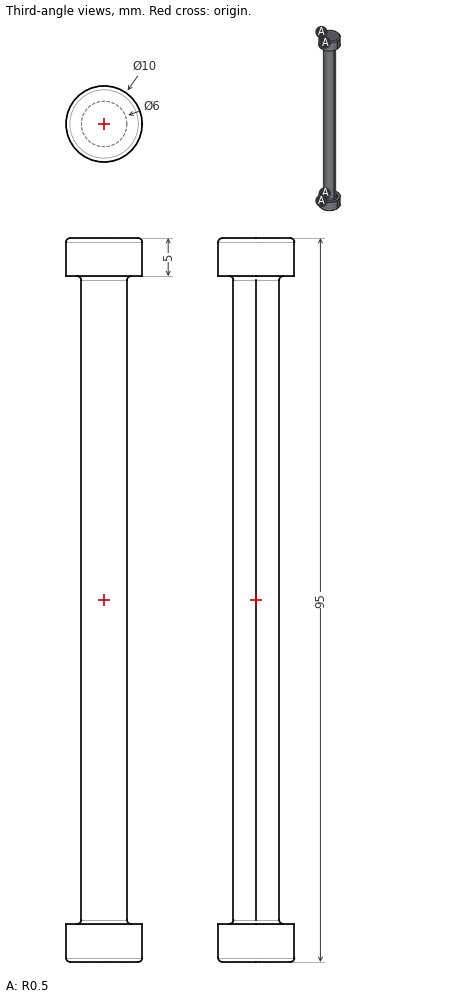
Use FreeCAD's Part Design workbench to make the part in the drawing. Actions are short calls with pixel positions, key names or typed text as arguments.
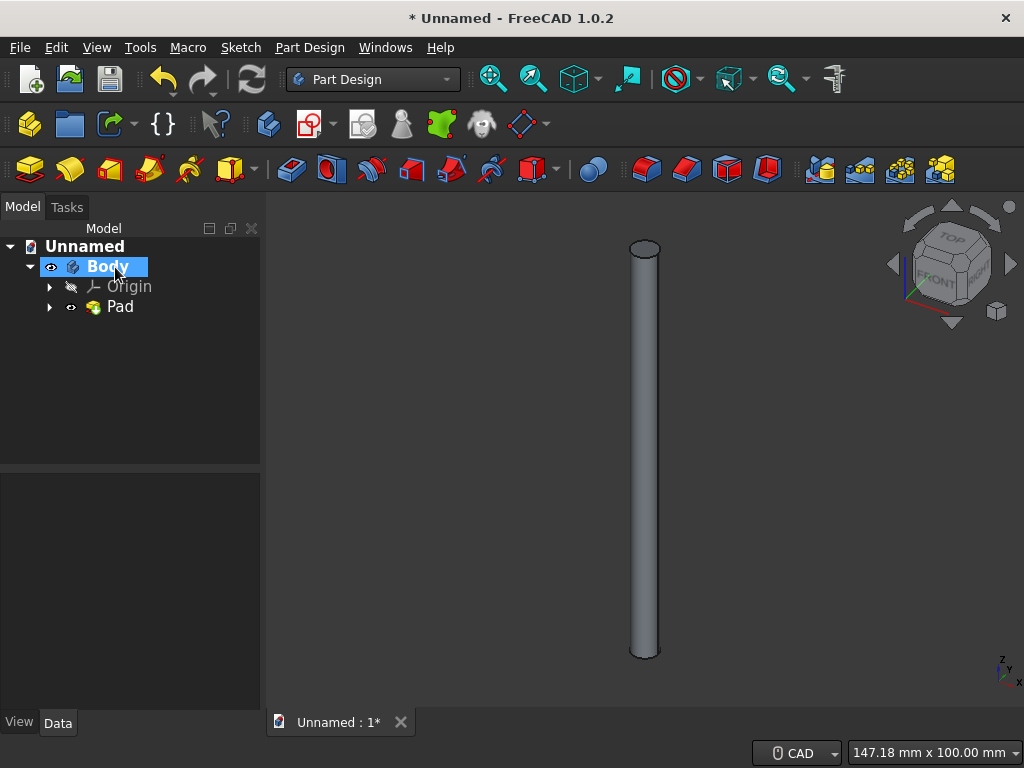
click(645, 248)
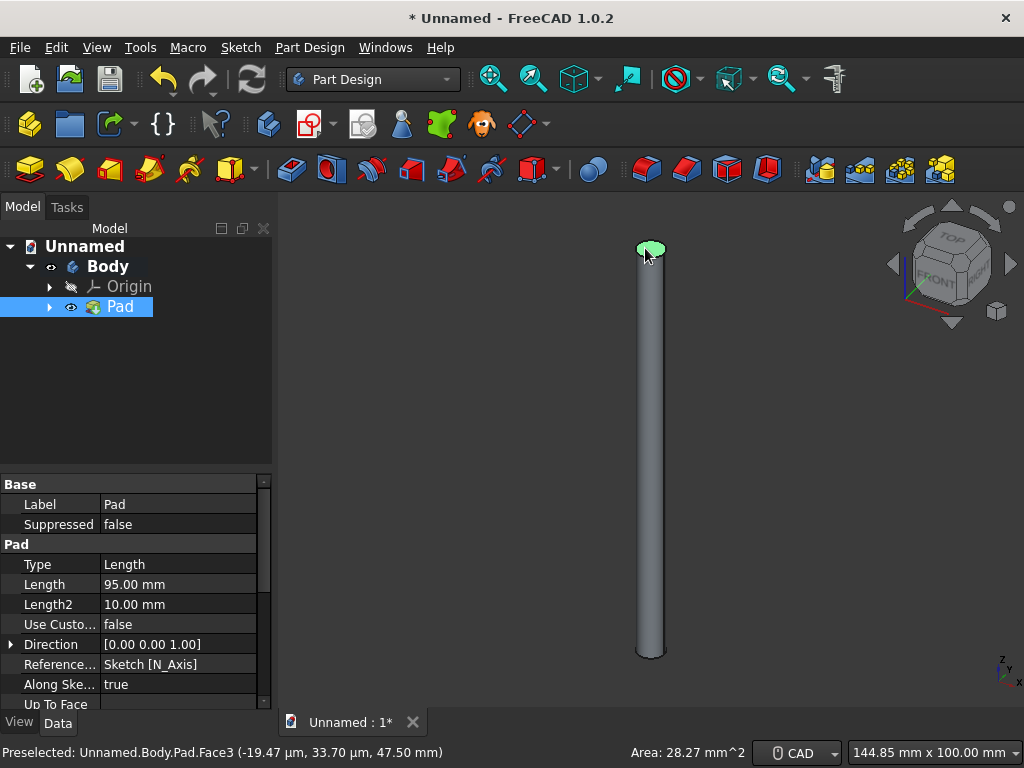
click(310, 124)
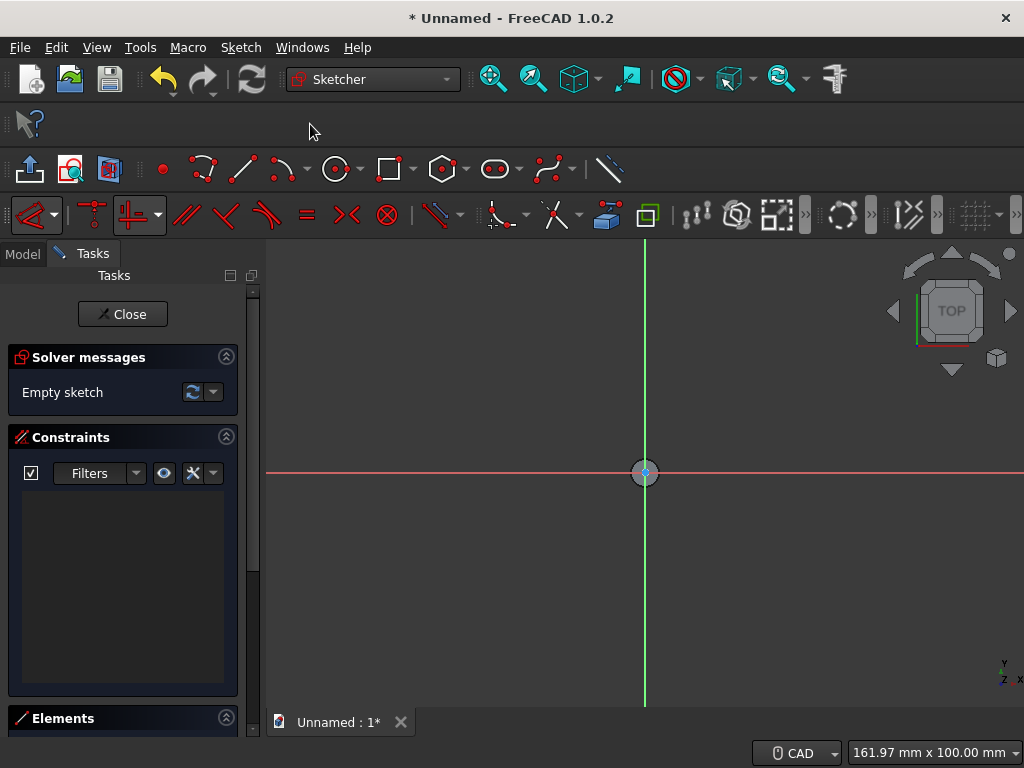
scroll(659, 473, up, 9)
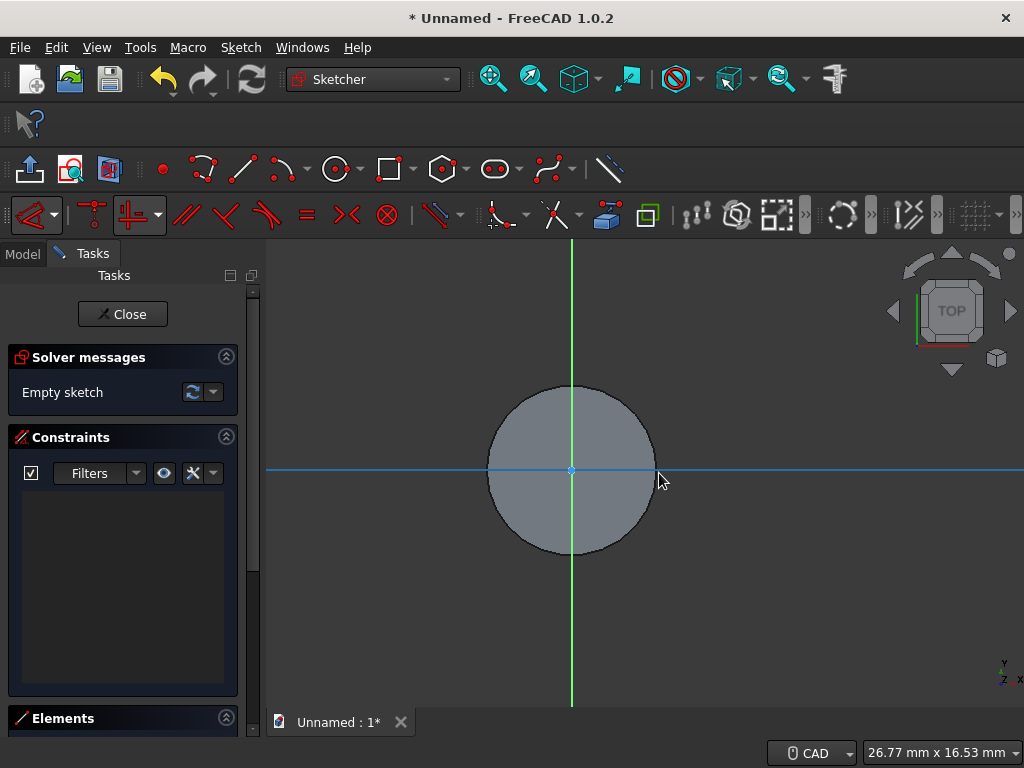
click(336, 170)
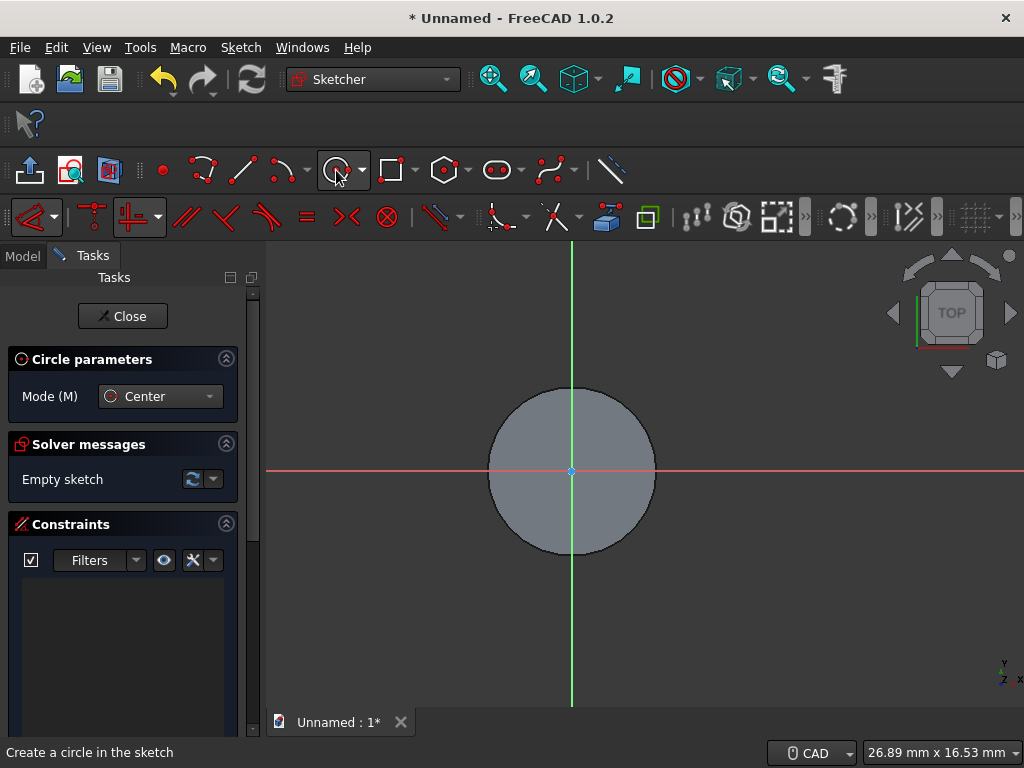
click(572, 471)
move(672, 372)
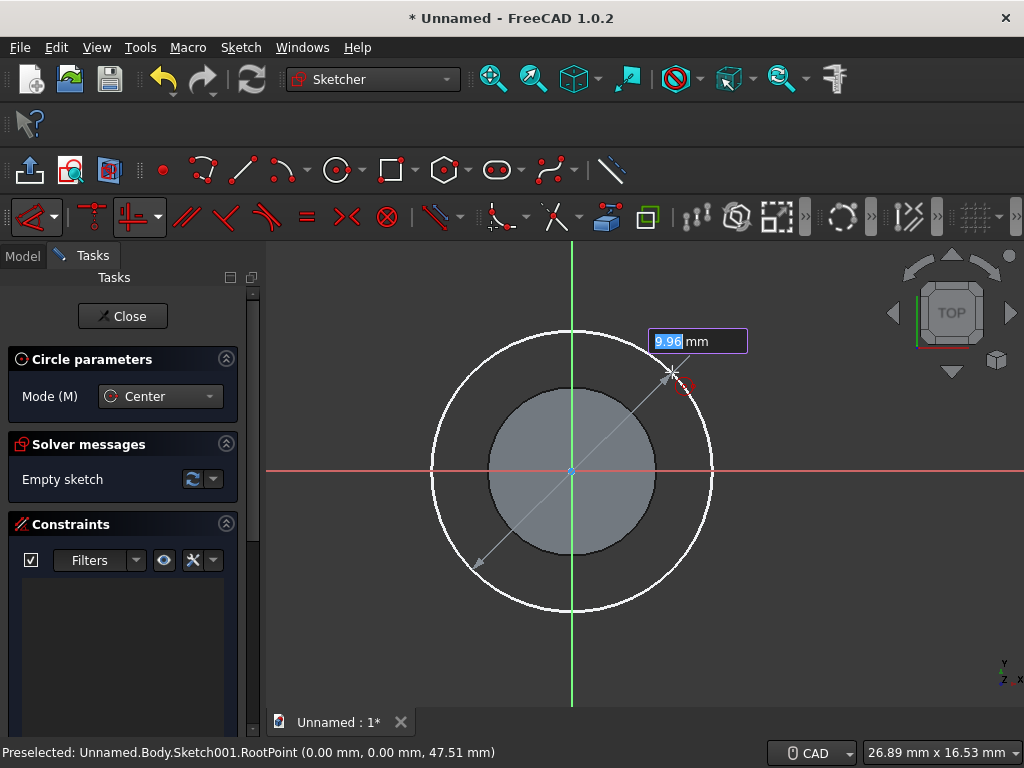
text(10)
key(Return)
key(Escape)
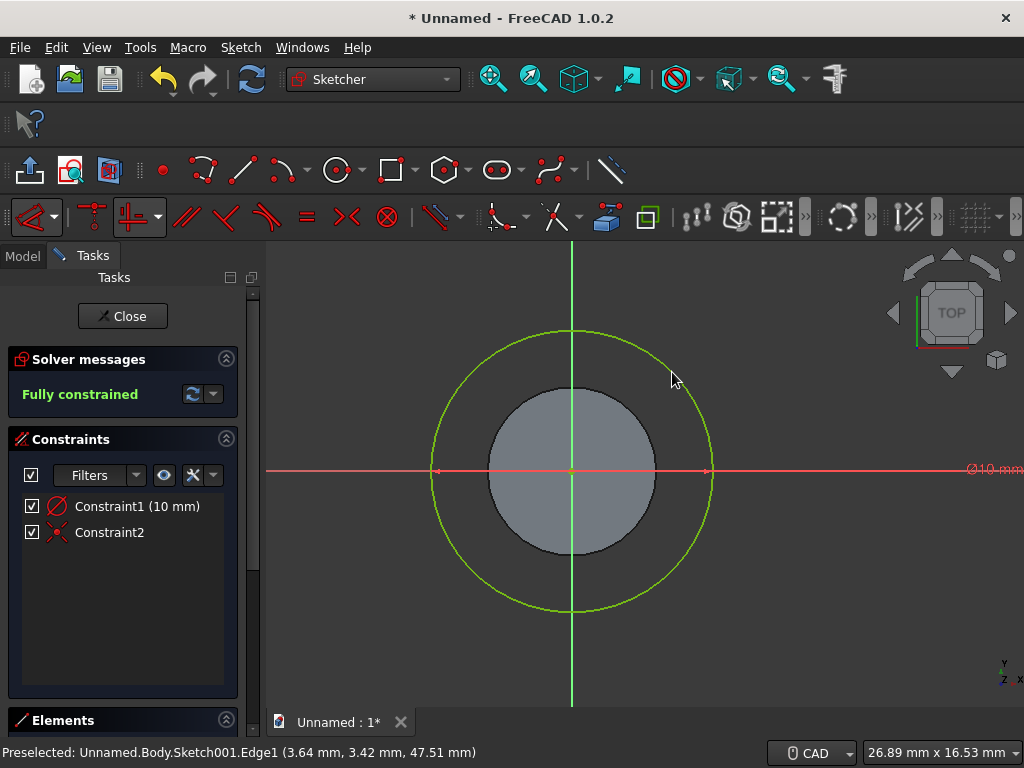
click(123, 316)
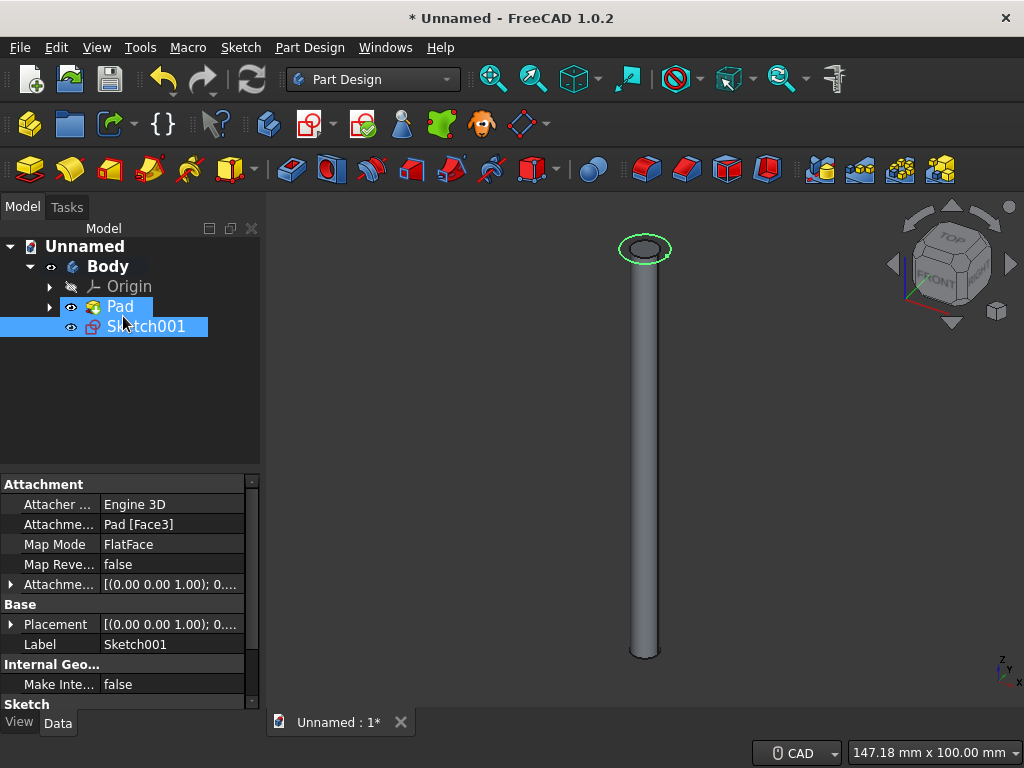
click(30, 170)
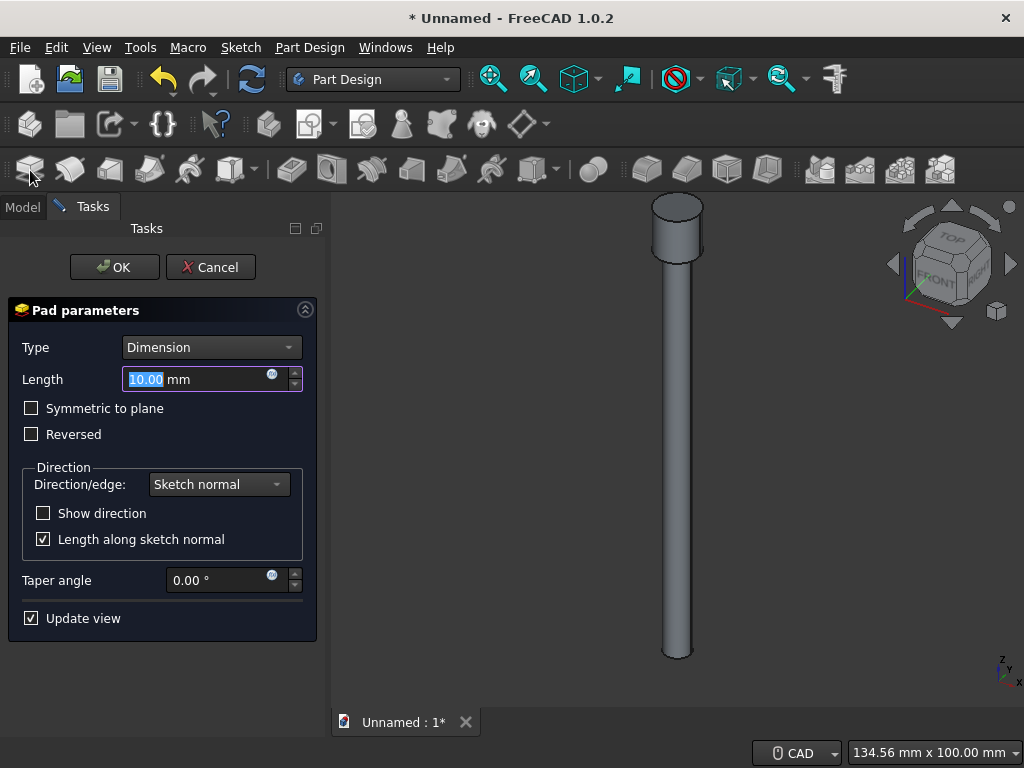
text(5)
key(Tab)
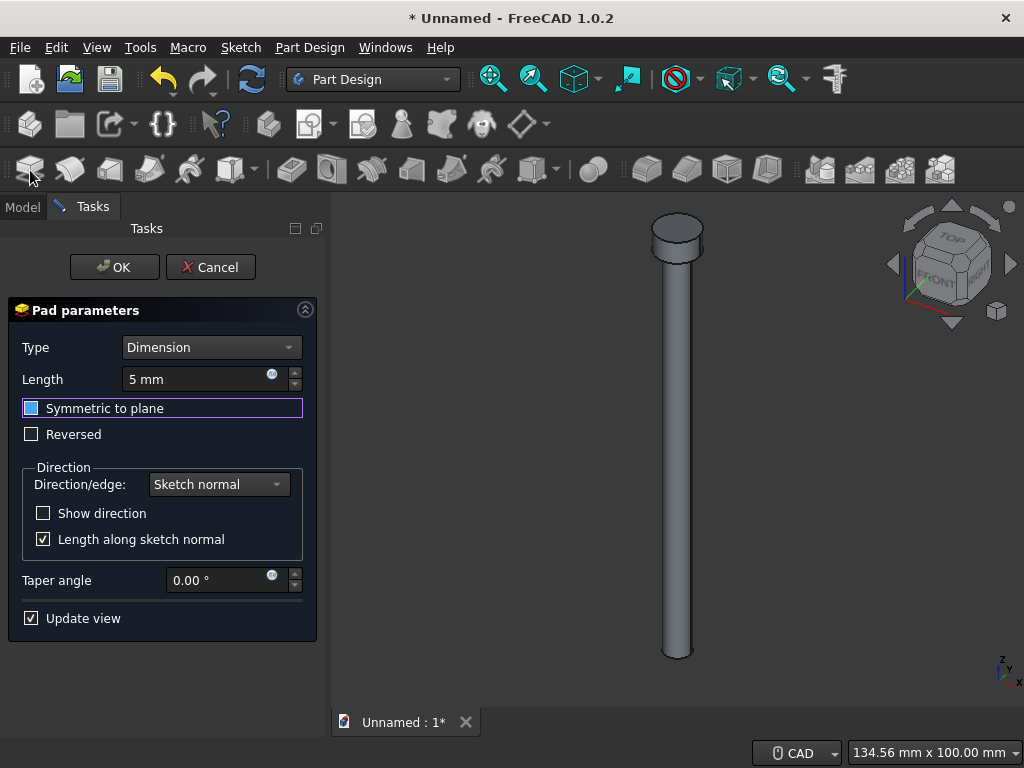
click(30, 434)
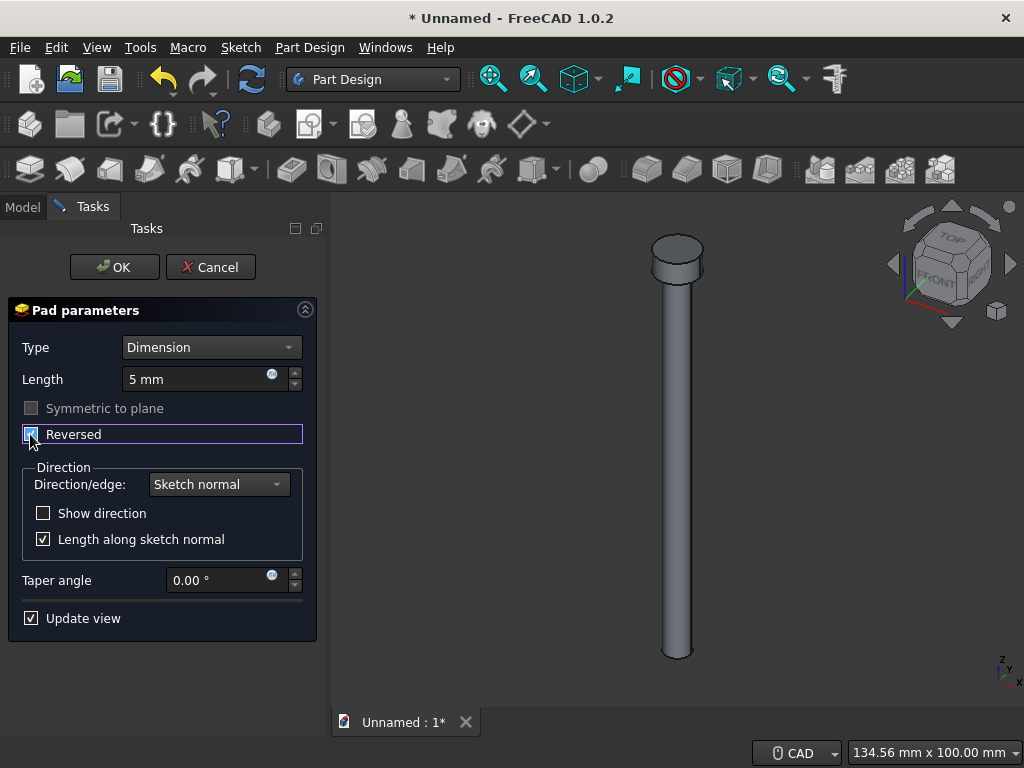
click(115, 267)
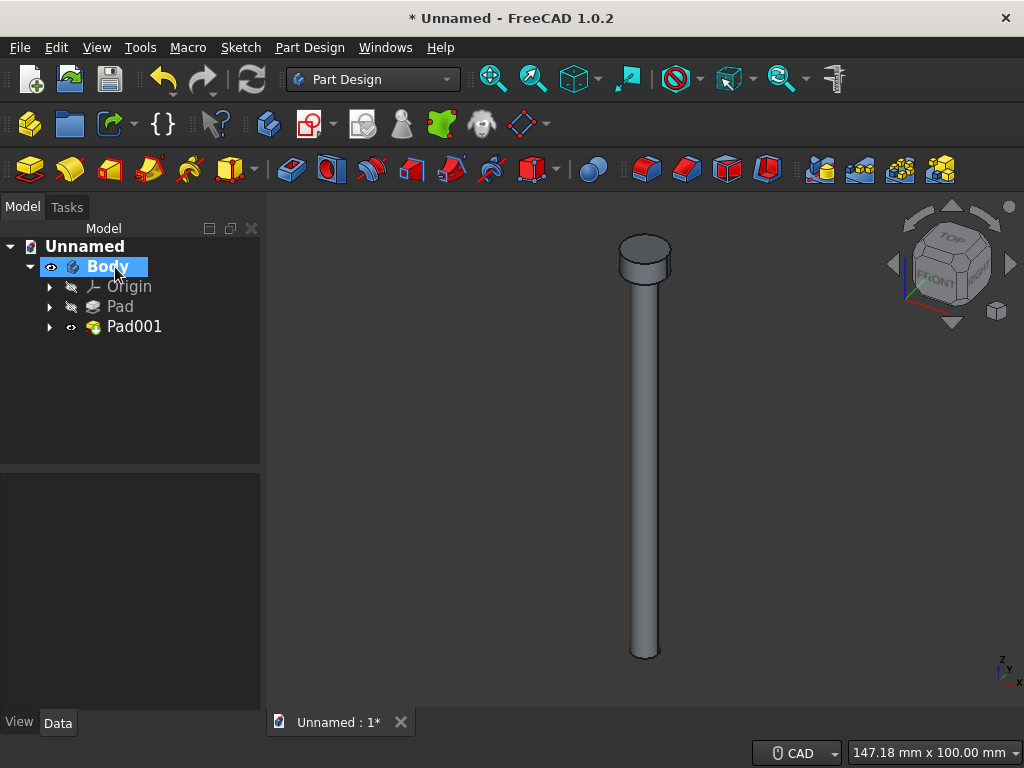
click(116, 327)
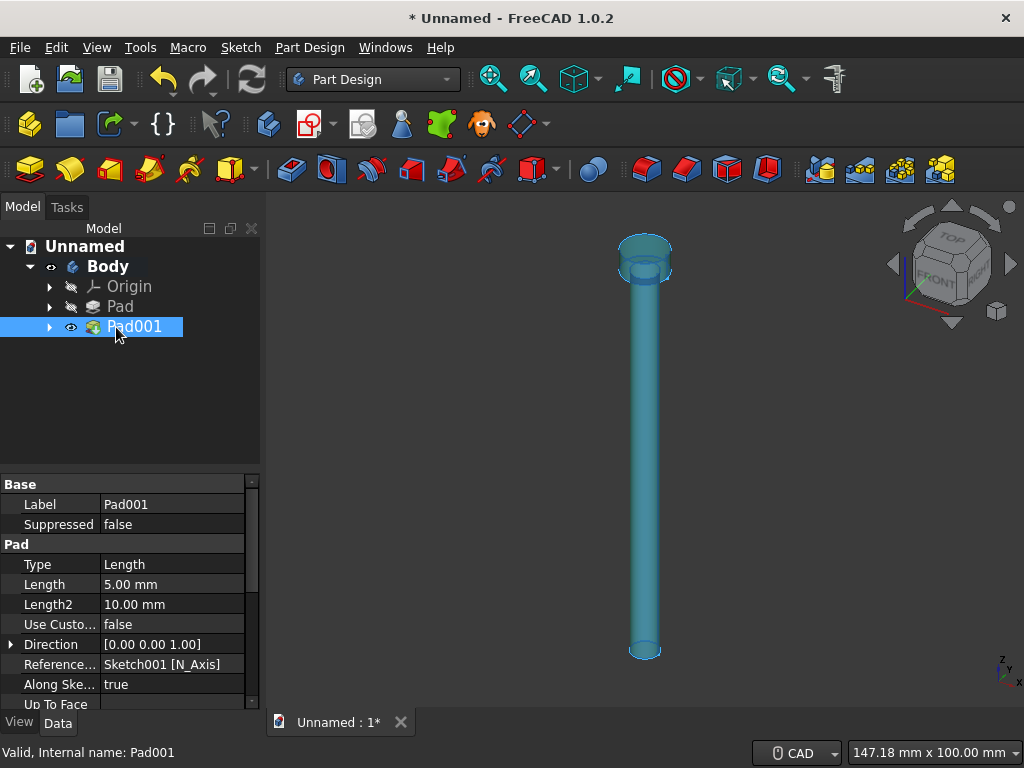
click(820, 170)